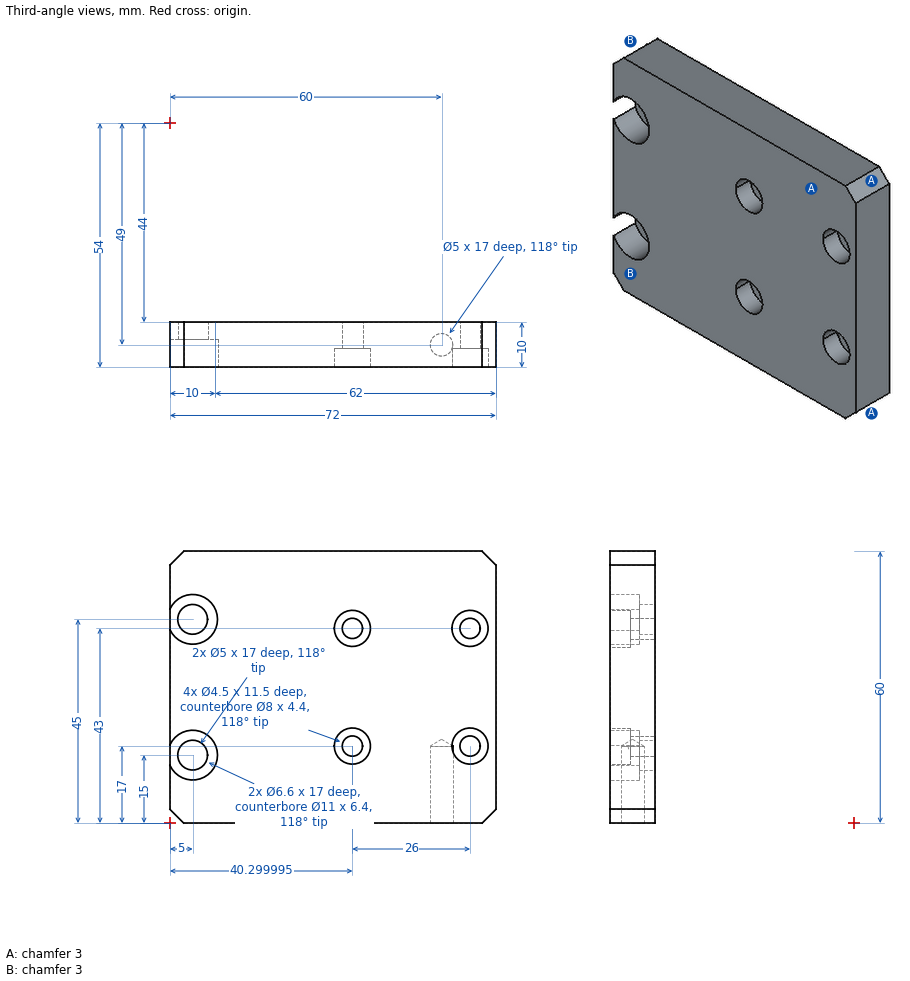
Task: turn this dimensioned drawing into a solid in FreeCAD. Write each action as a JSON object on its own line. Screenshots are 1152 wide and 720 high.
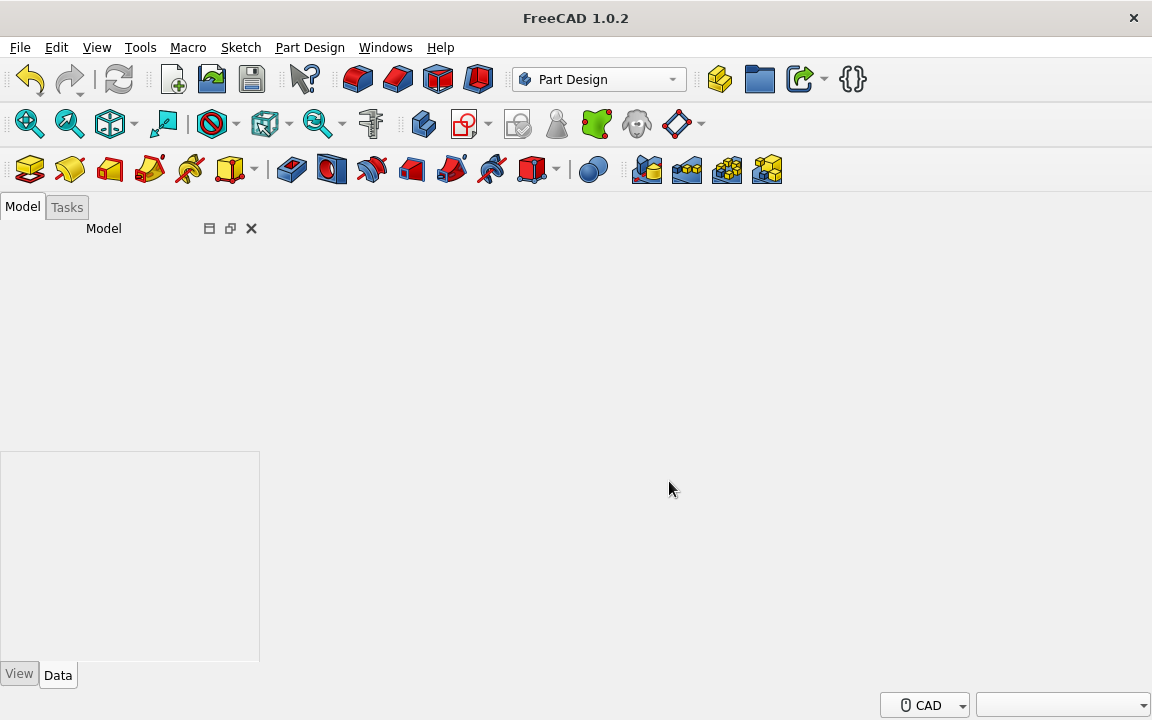
{"action": "left_click", "coordinate": [172, 80]}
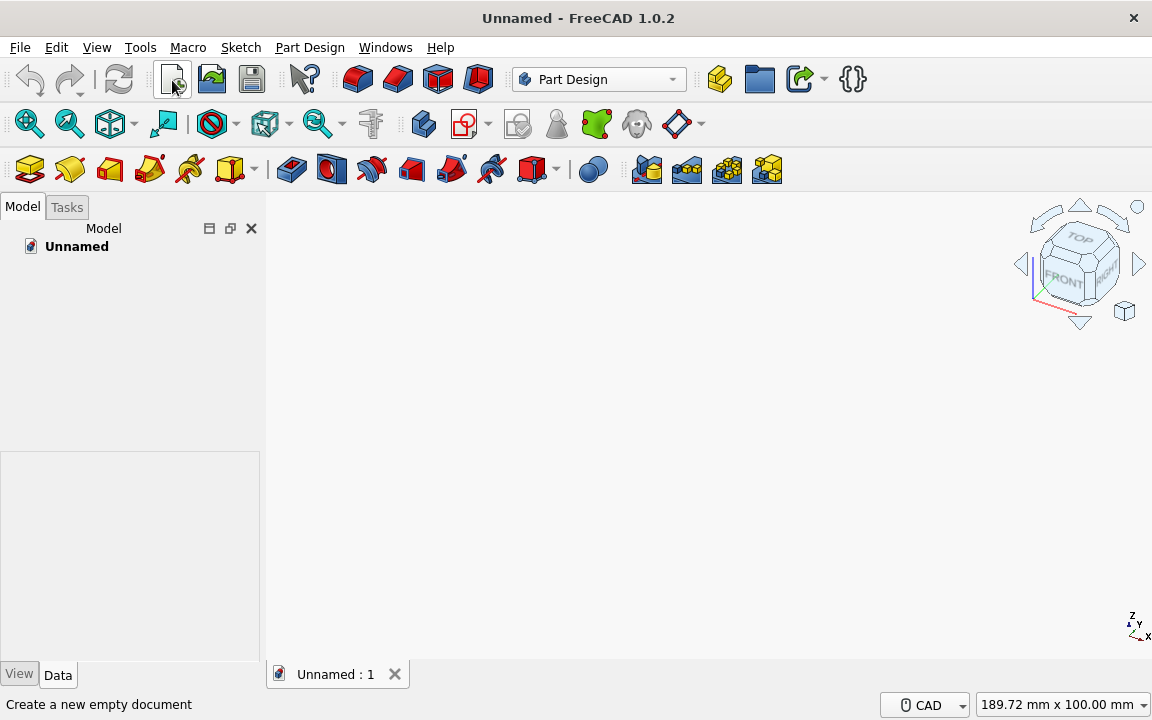
{"action": "left_click", "coordinate": [464, 124]}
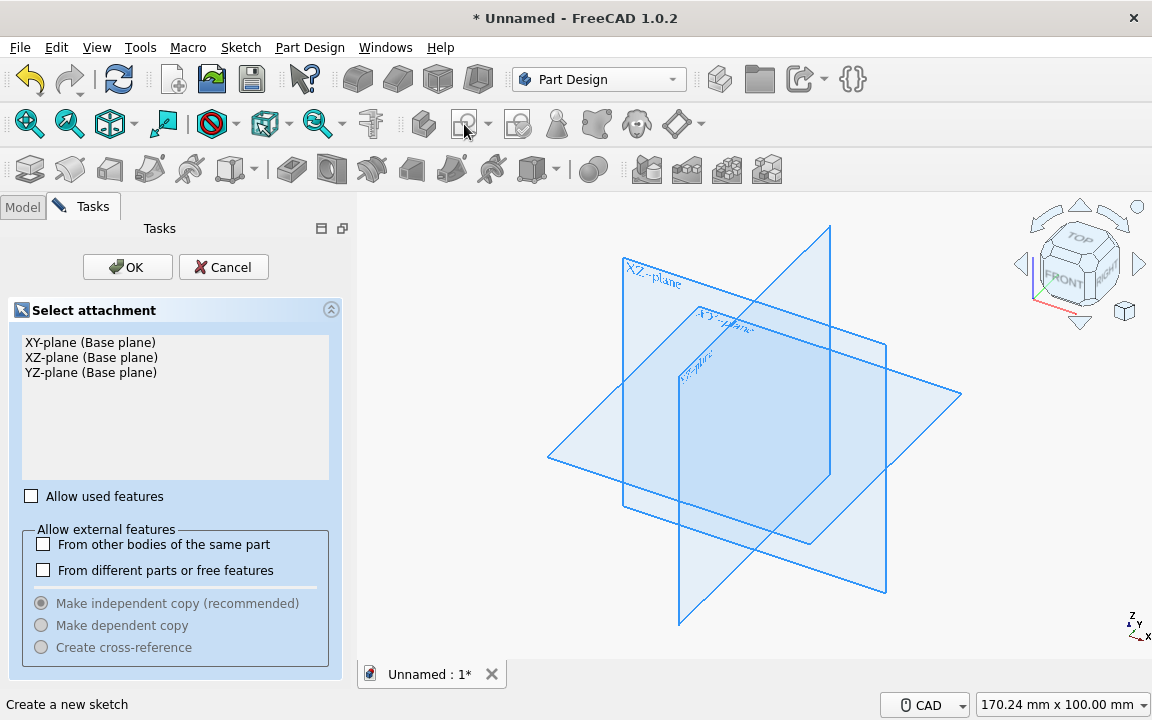
{"action": "left_click", "coordinate": [82, 342]}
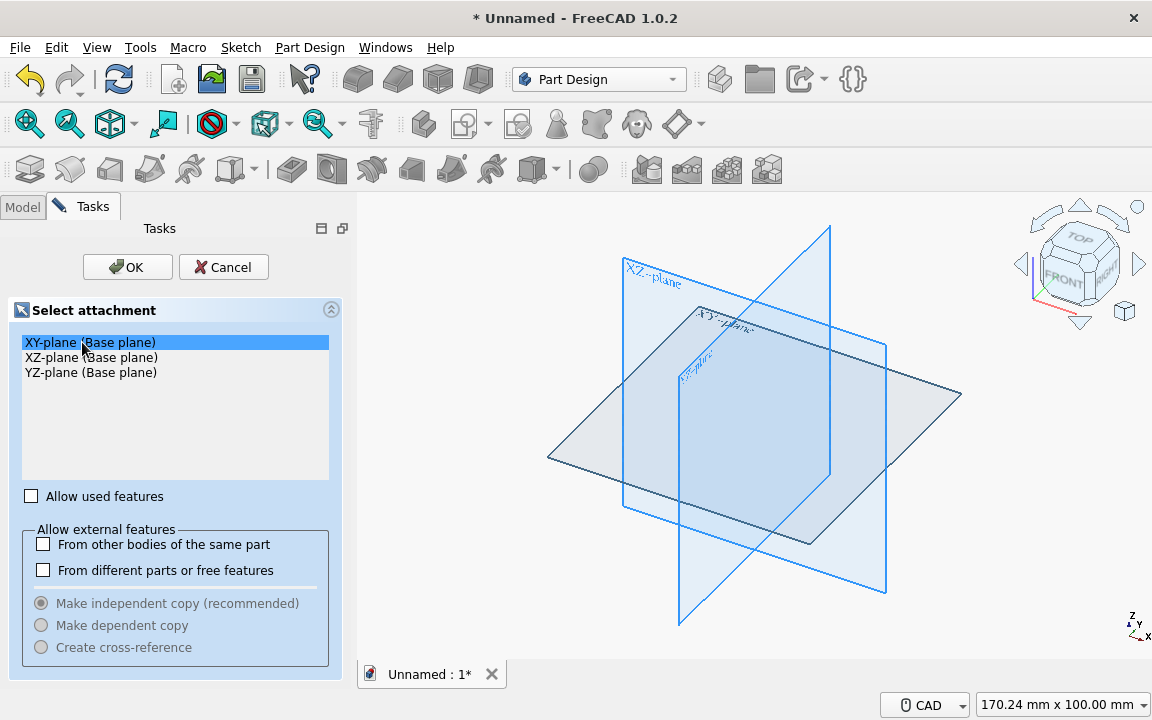
{"action": "left_click", "coordinate": [128, 267]}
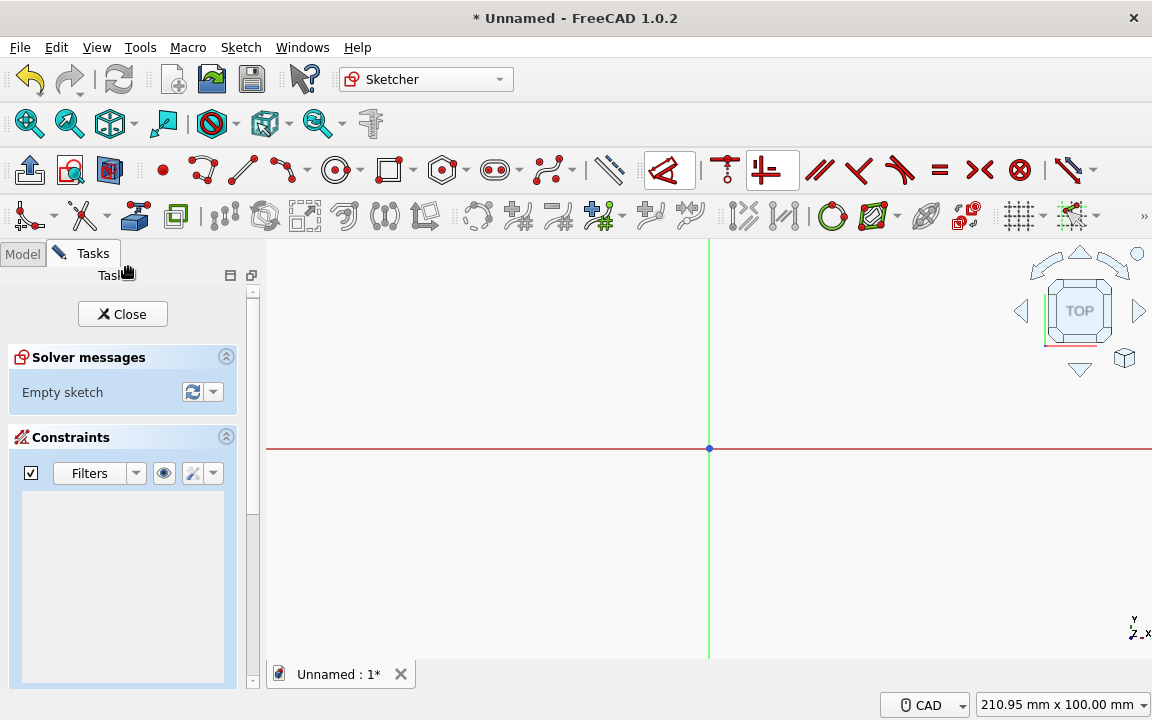
{"action": "scroll", "coordinate": [294, 267], "scroll_direction": "down", "scroll_amount": 1}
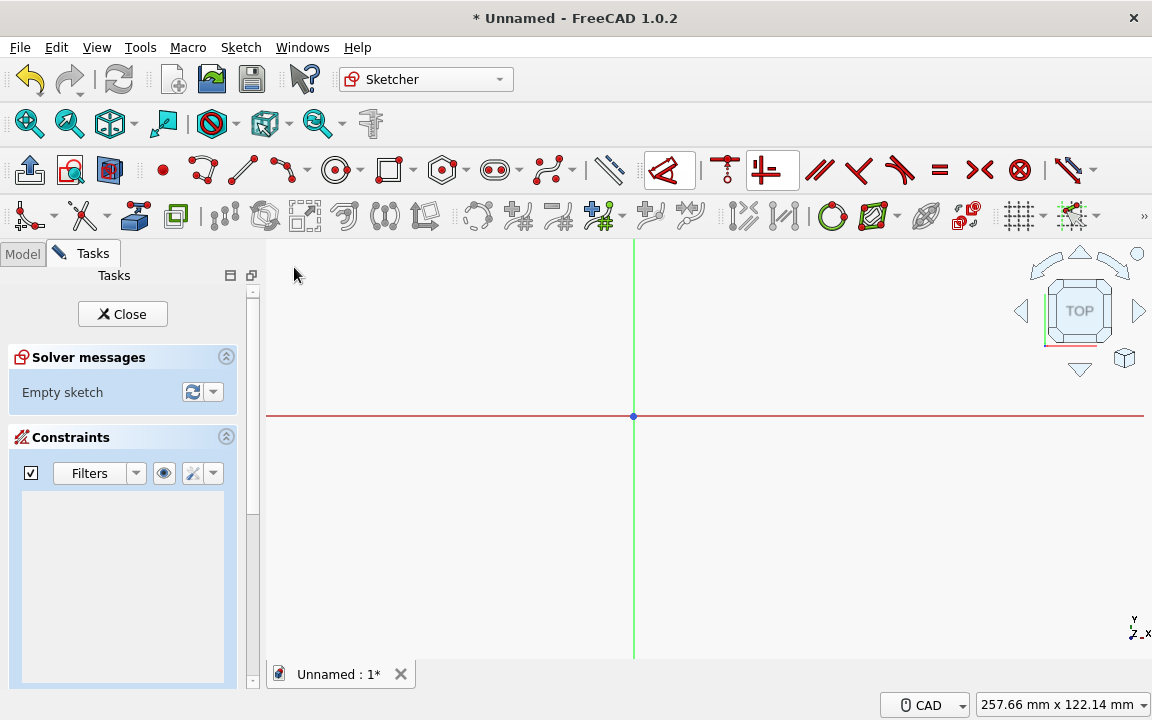
{"action": "scroll", "coordinate": [987, 631], "scroll_direction": "up", "scroll_amount": 2}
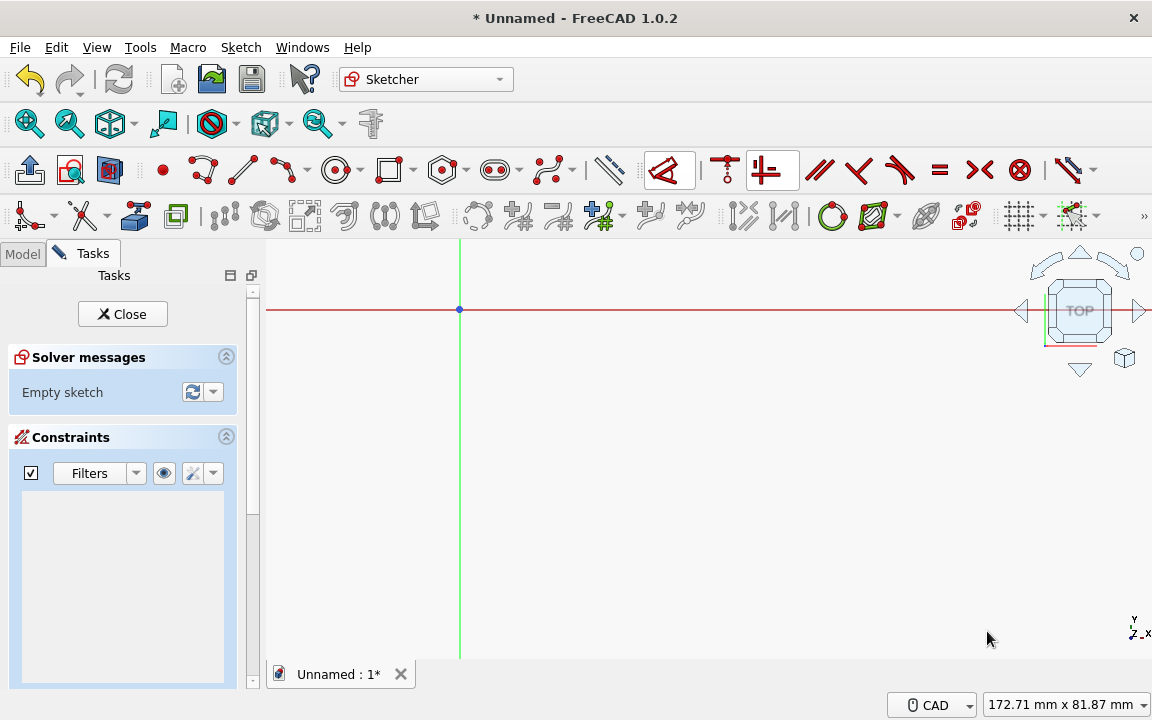
{"action": "left_click", "coordinate": [204, 170]}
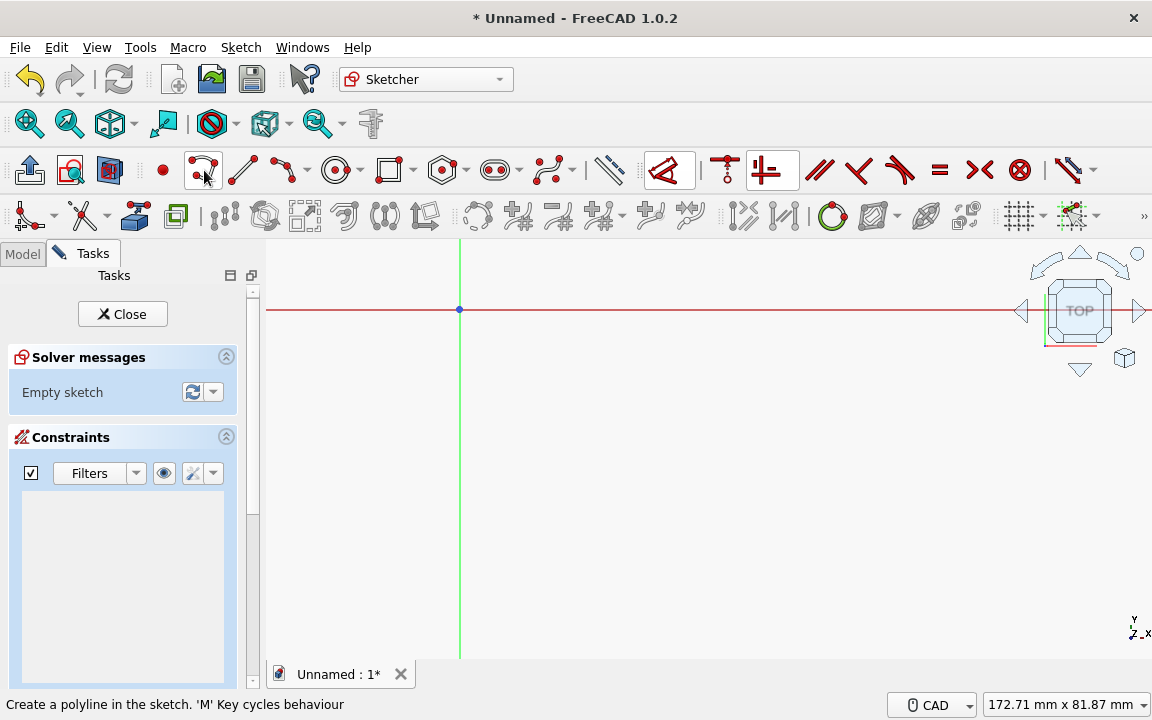
{"action": "left_click", "coordinate": [460, 310]}
{"action": "left_click", "coordinate": [469, 587]}
{"action": "left_click", "coordinate": [829, 587]}
{"action": "left_click", "coordinate": [829, 536]}
{"action": "left_click", "coordinate": [511, 536]}
{"action": "left_click", "coordinate": [511, 319]}
{"action": "left_click", "coordinate": [460, 310]}
{"action": "key", "text": "Escape"}
{"action": "key", "text": "Escape"}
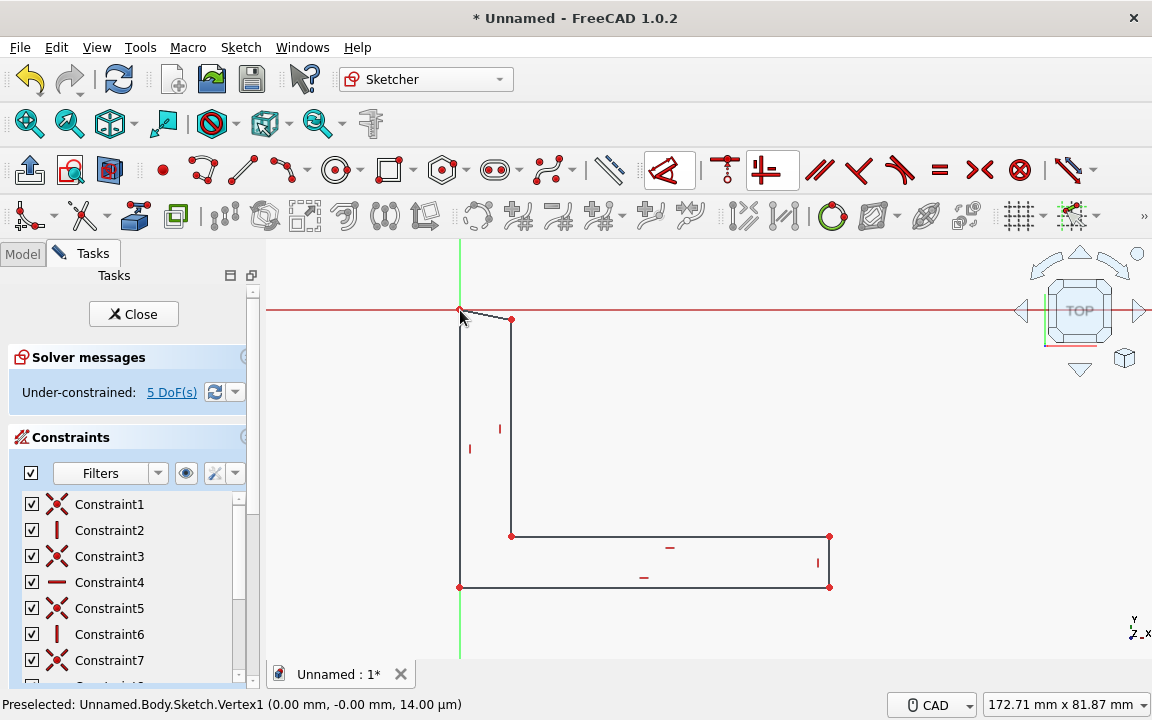
{"action": "left_click", "coordinate": [475, 313]}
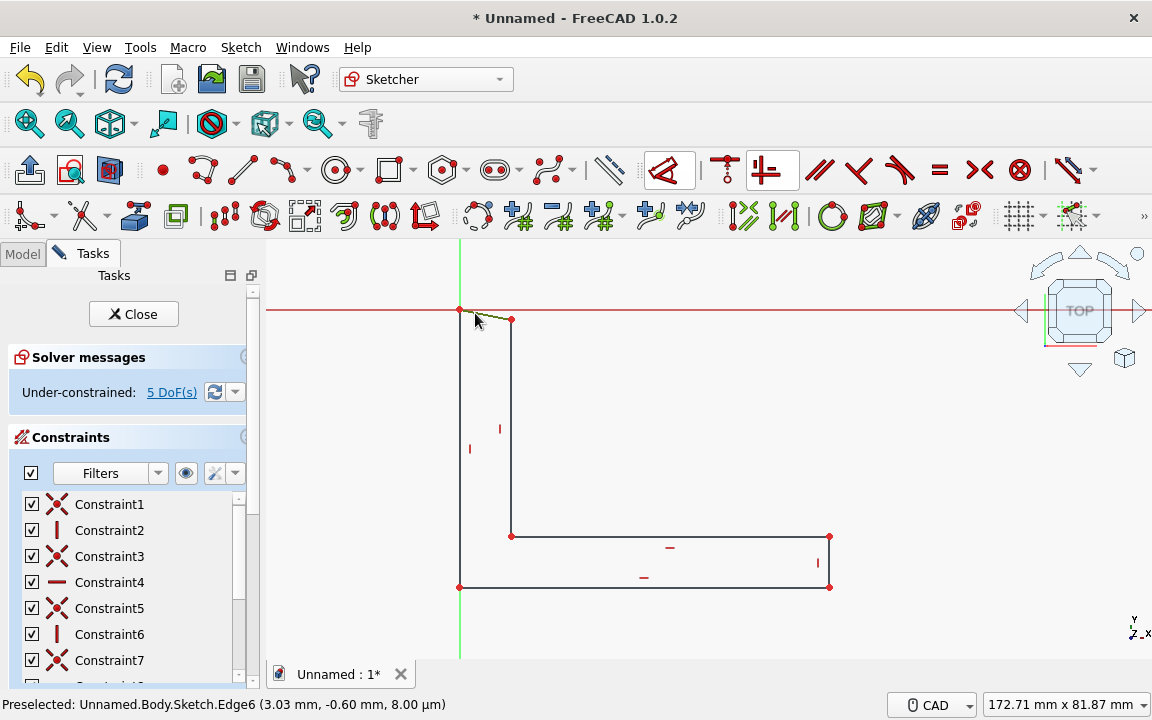
{"action": "left_click", "coordinate": [794, 170]}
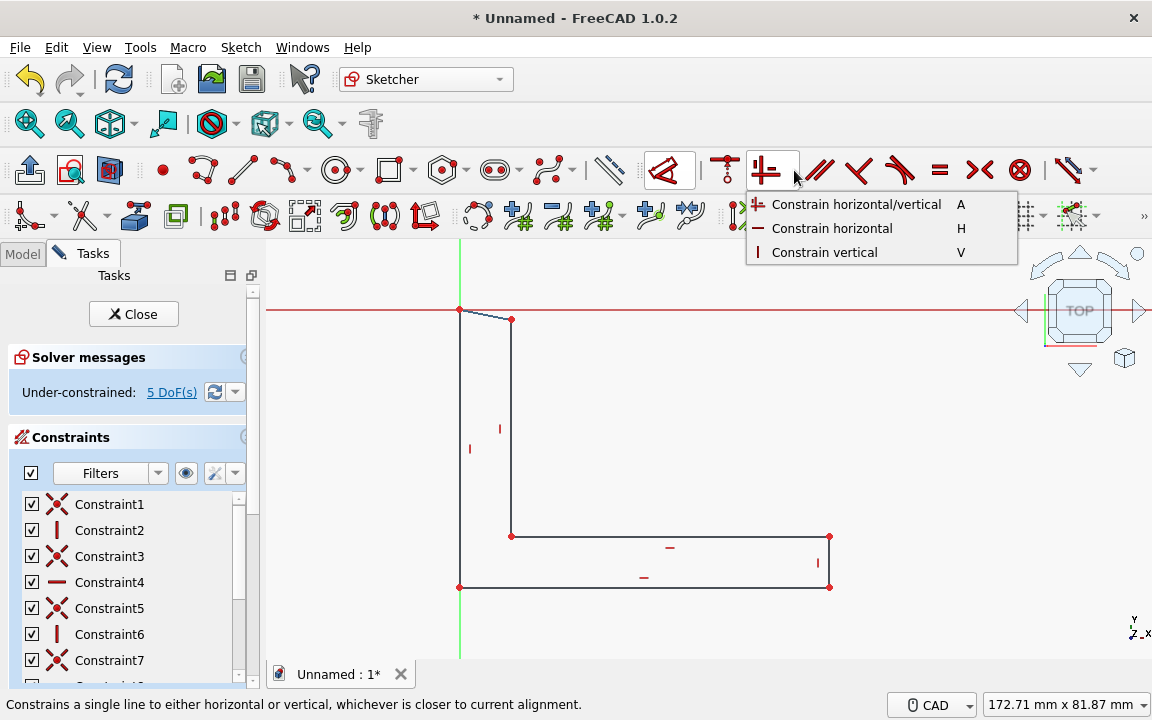
{"action": "left_click", "coordinate": [882, 228]}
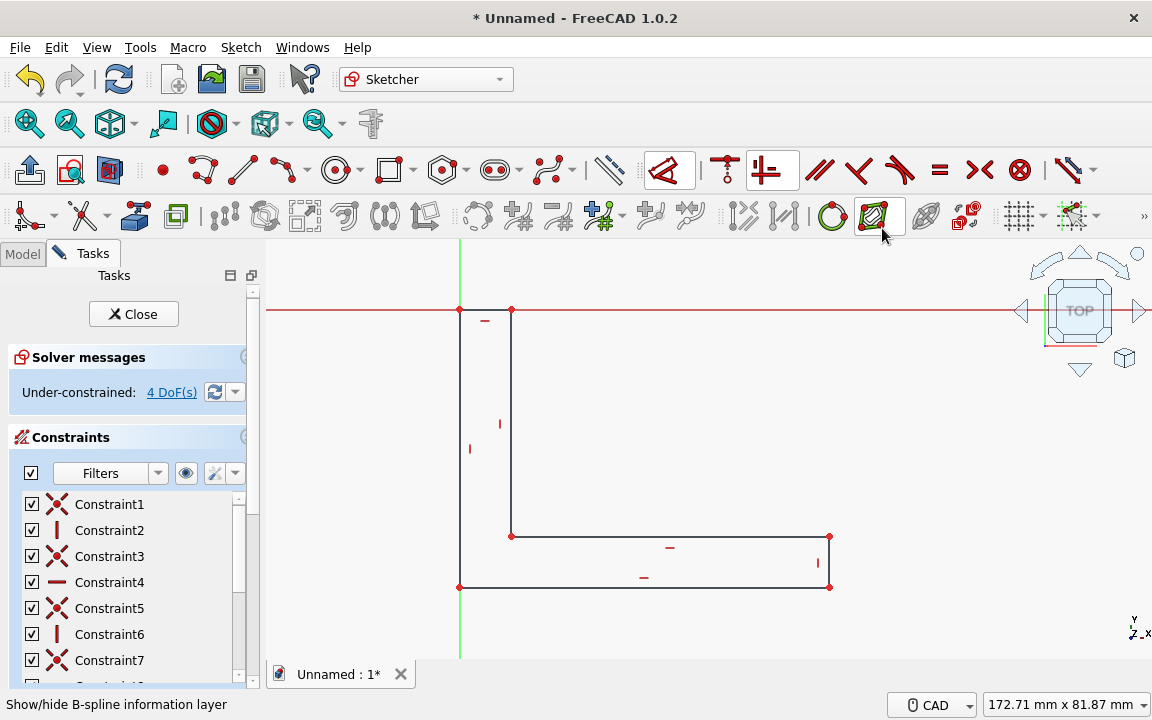
{"action": "left_click", "coordinate": [664, 170]}